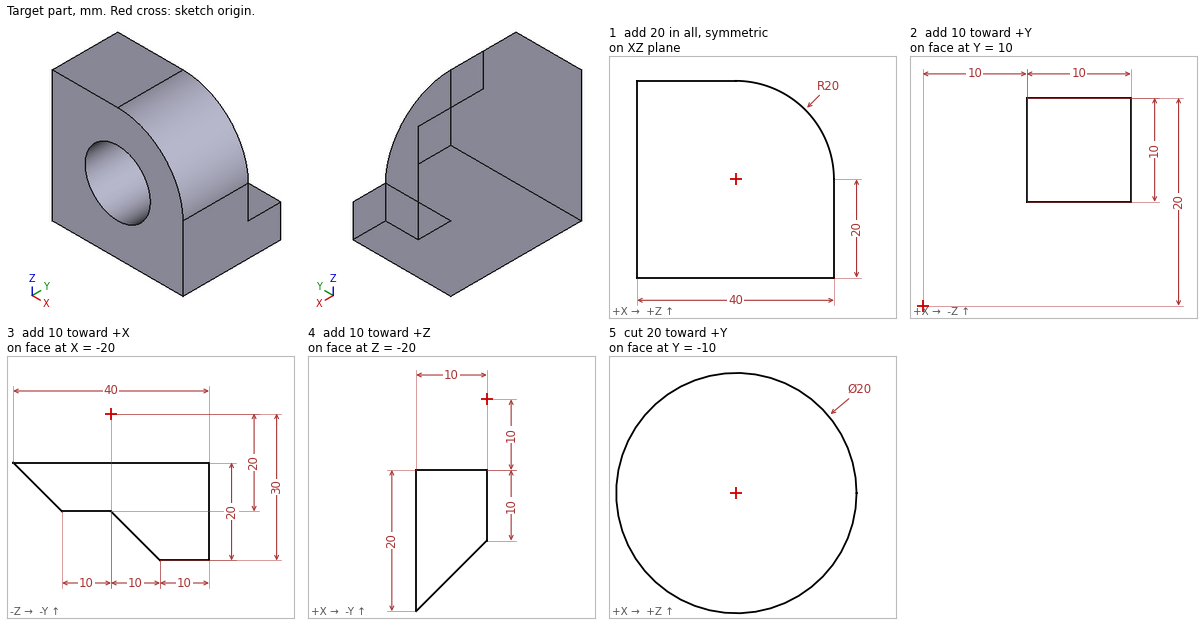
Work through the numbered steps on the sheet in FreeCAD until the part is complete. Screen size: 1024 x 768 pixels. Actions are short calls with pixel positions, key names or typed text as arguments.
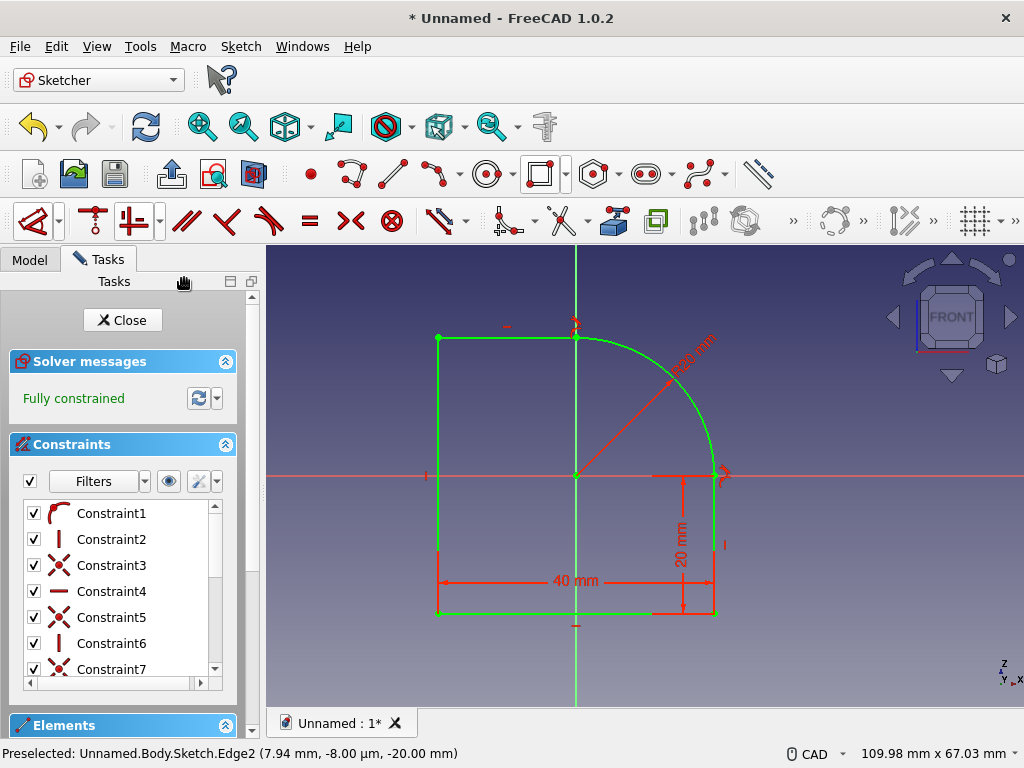
click(123, 320)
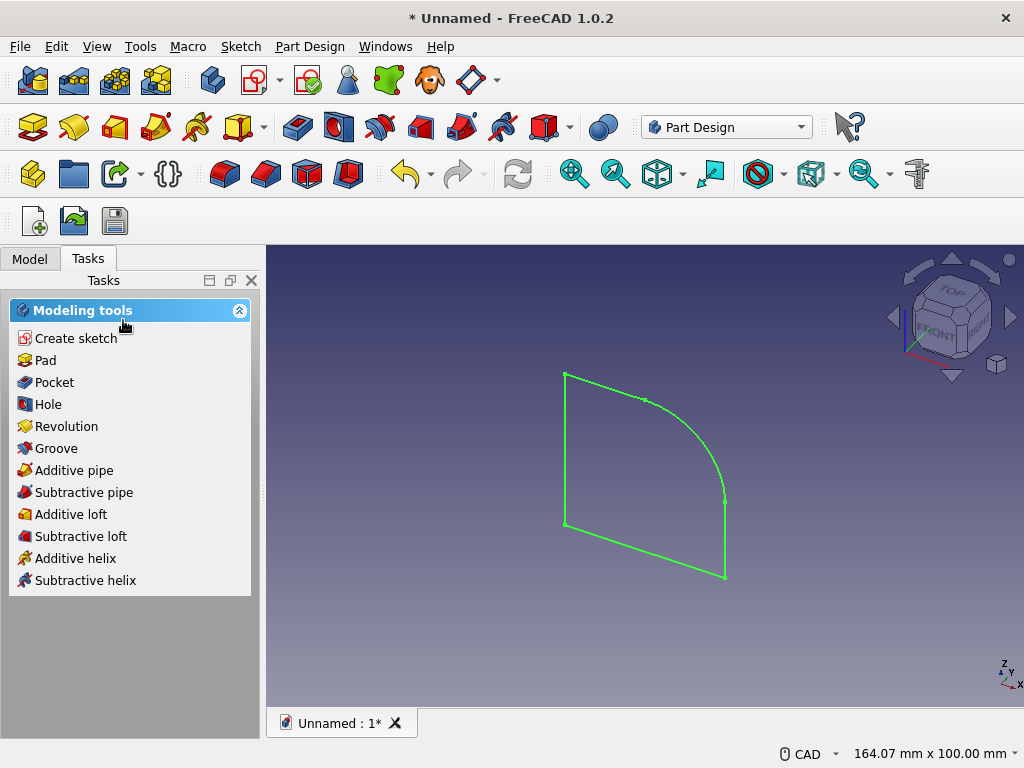
click(33, 128)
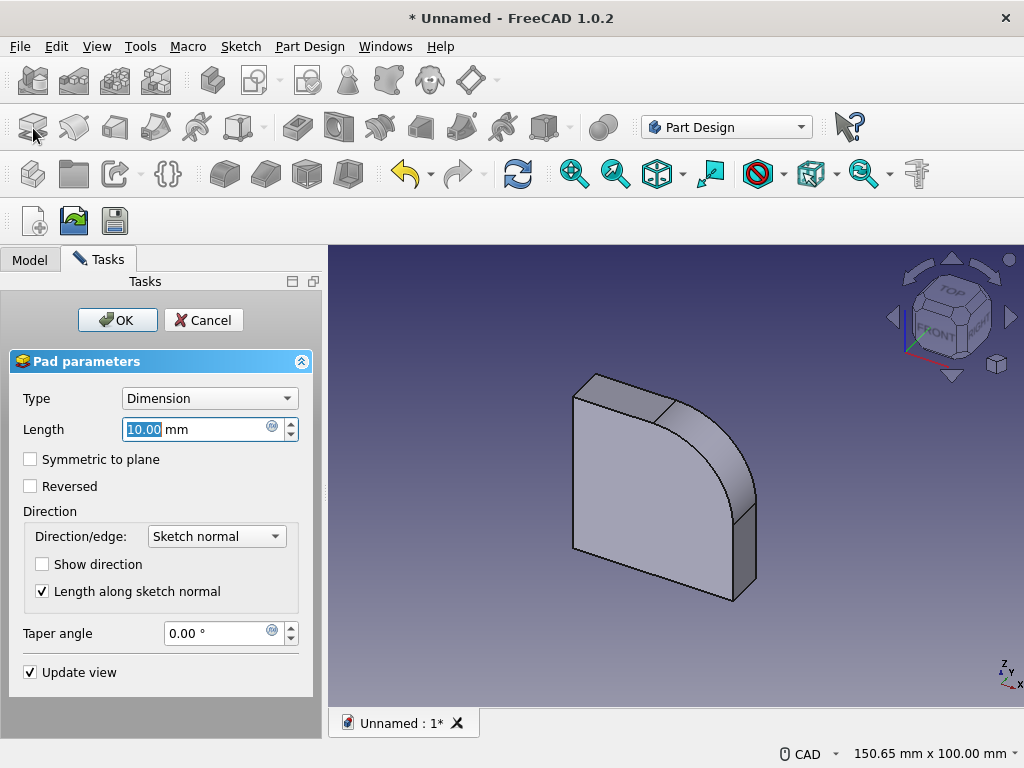
text(20)
key(Tab)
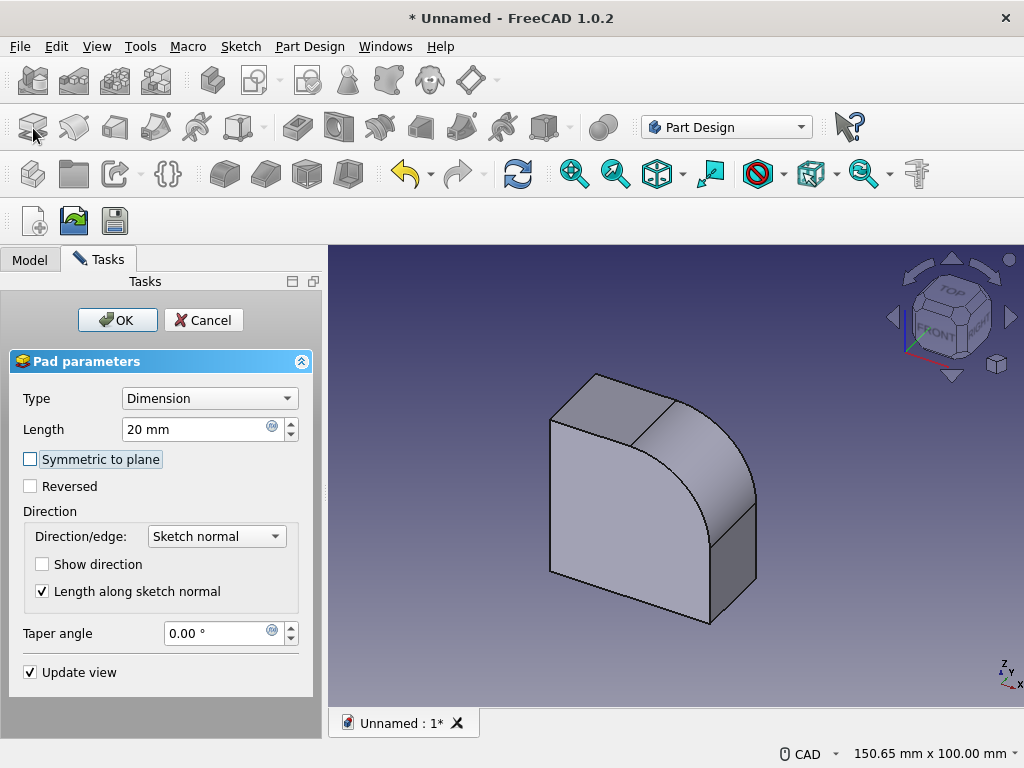
click(31, 459)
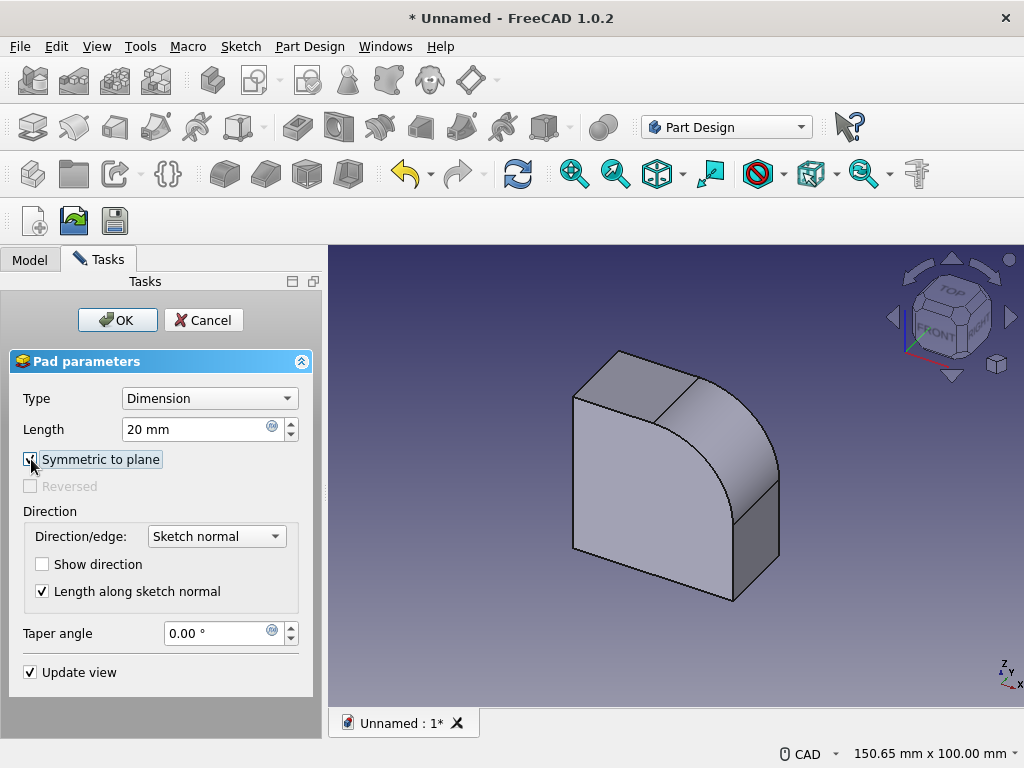
click(118, 320)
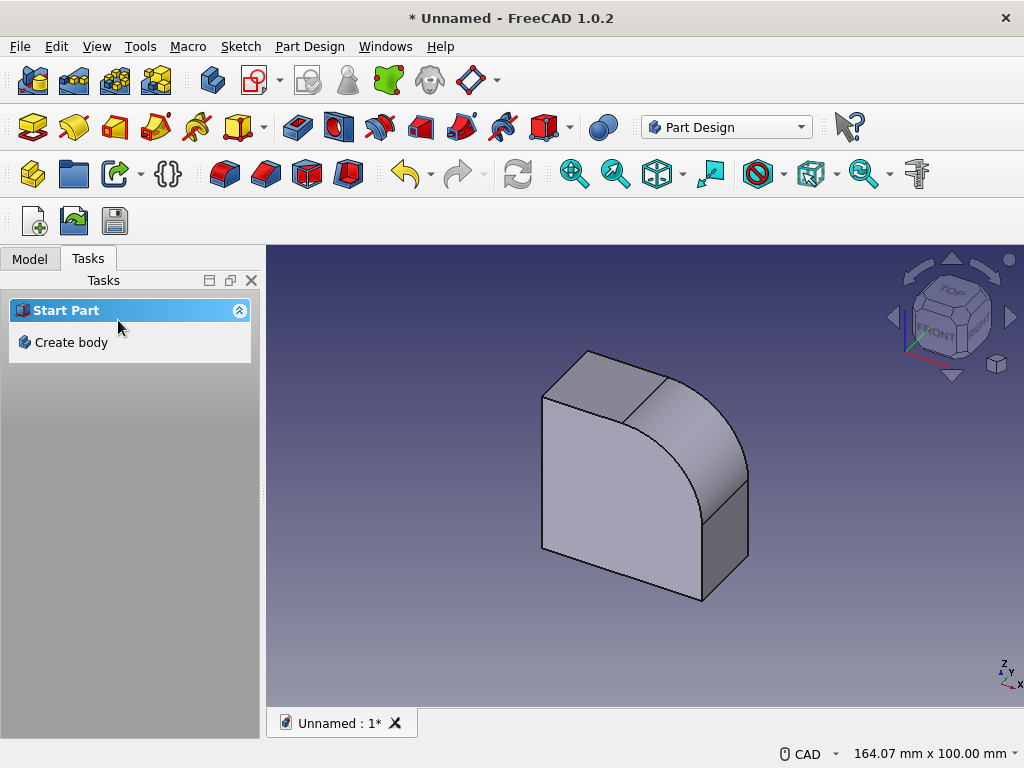
key(4)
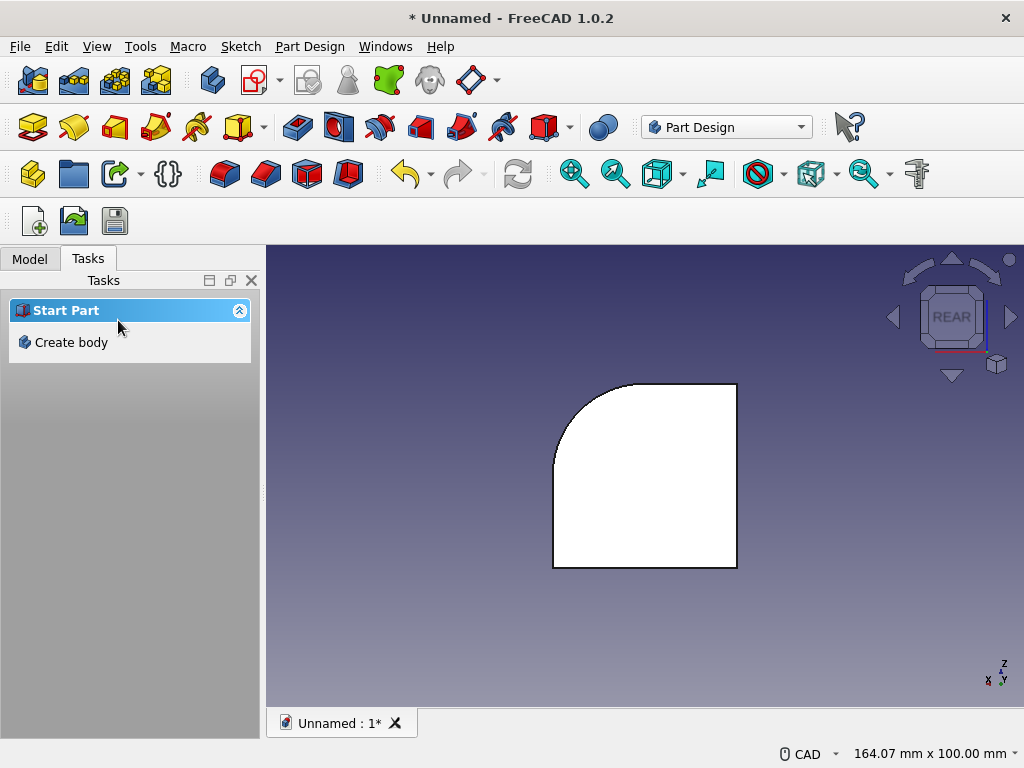
click(575, 174)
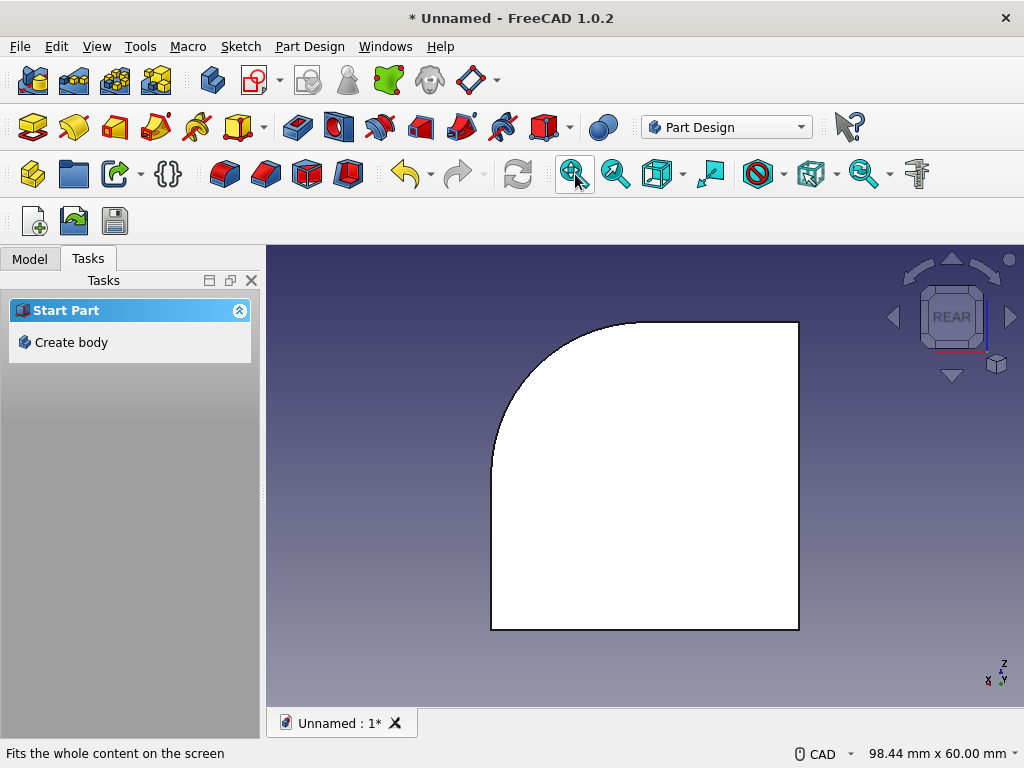
click(645, 475)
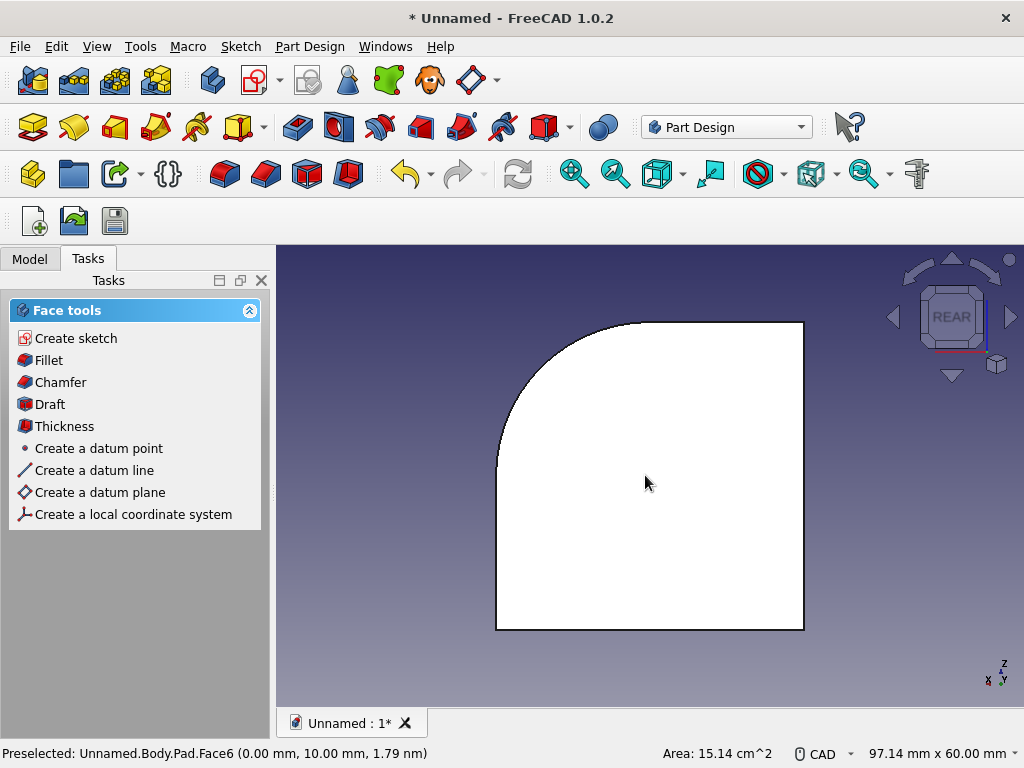
click(254, 80)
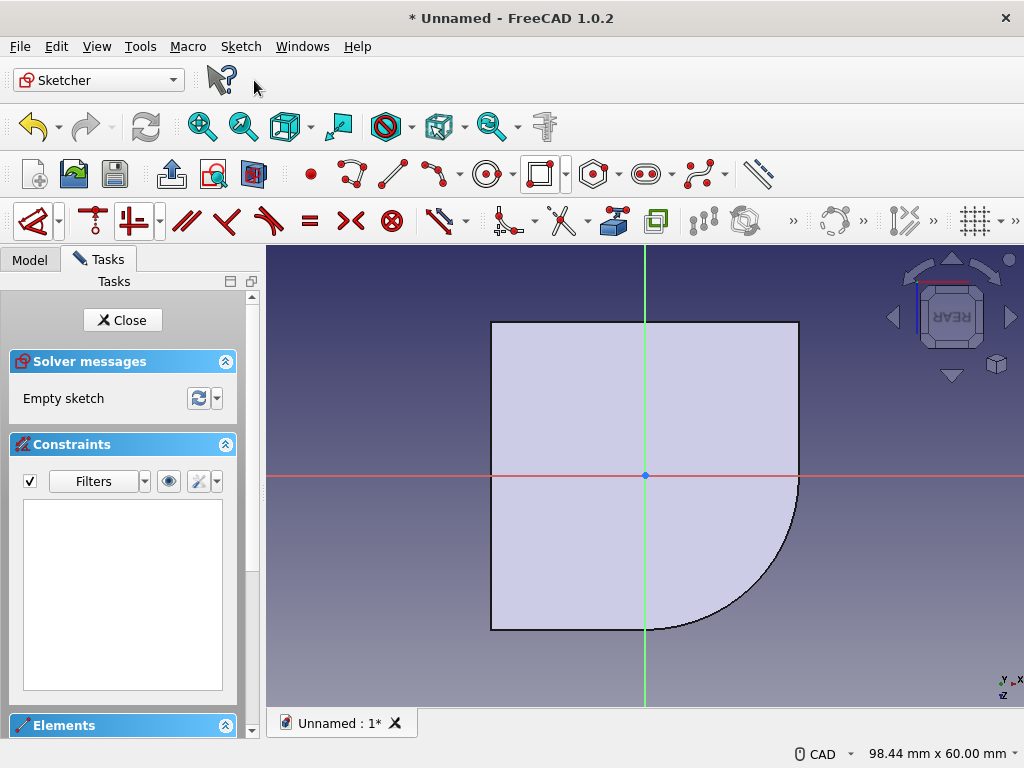
scroll(859, 305, up, 3)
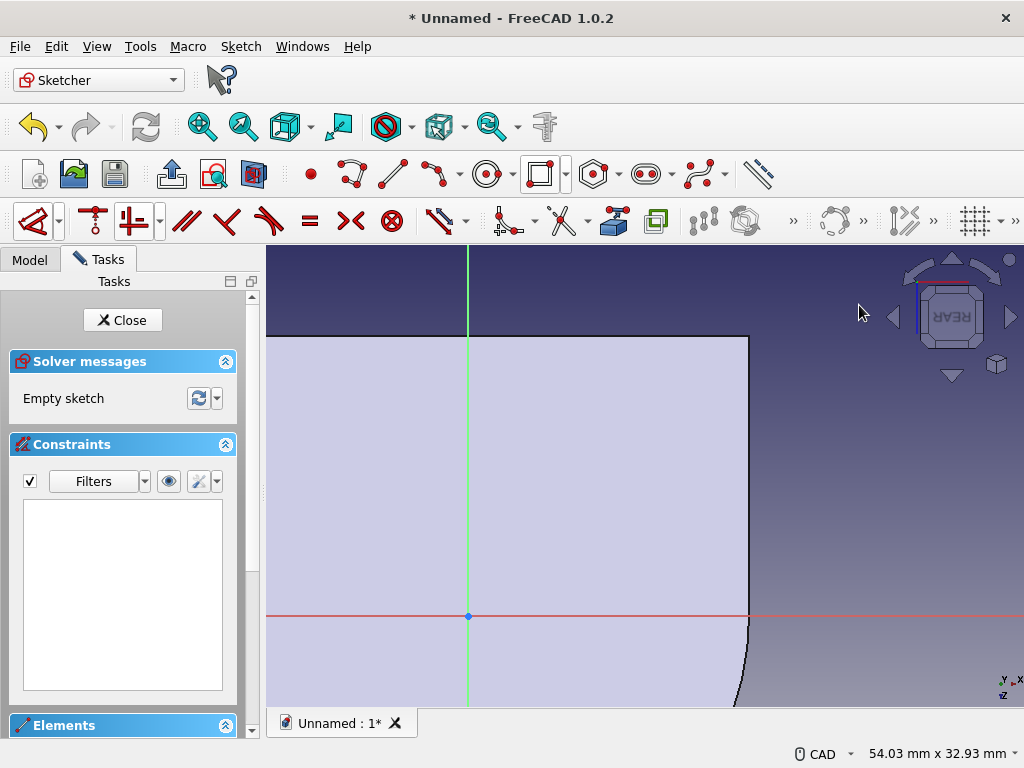
click(540, 174)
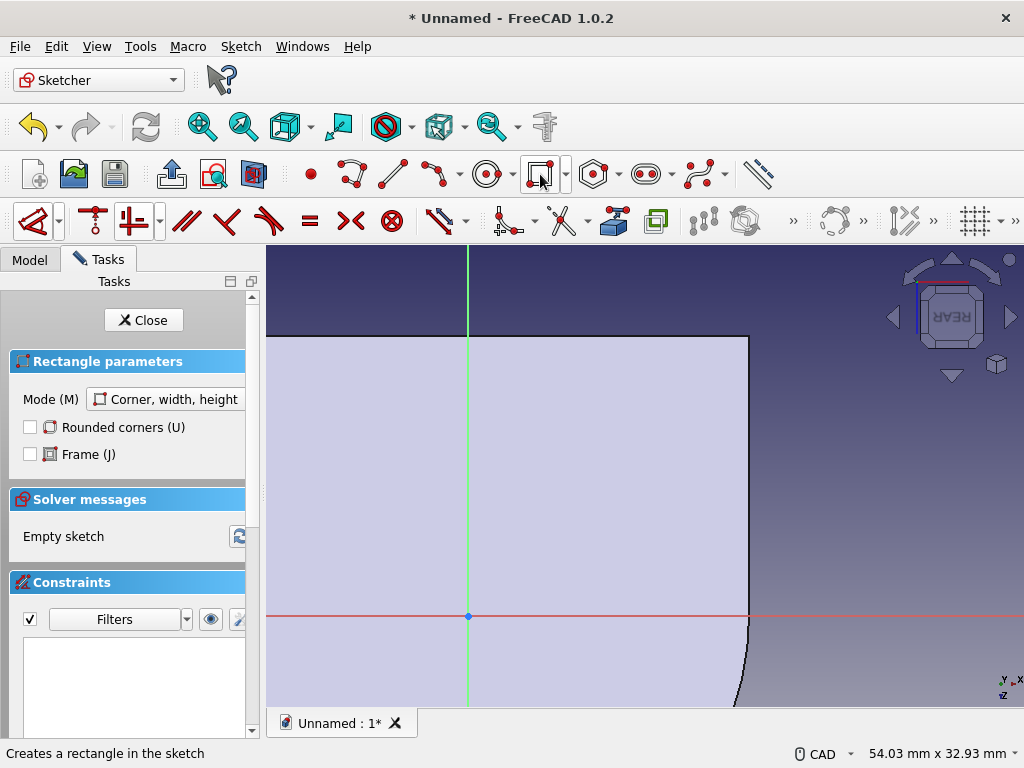
click(609, 336)
click(749, 476)
key(Escape)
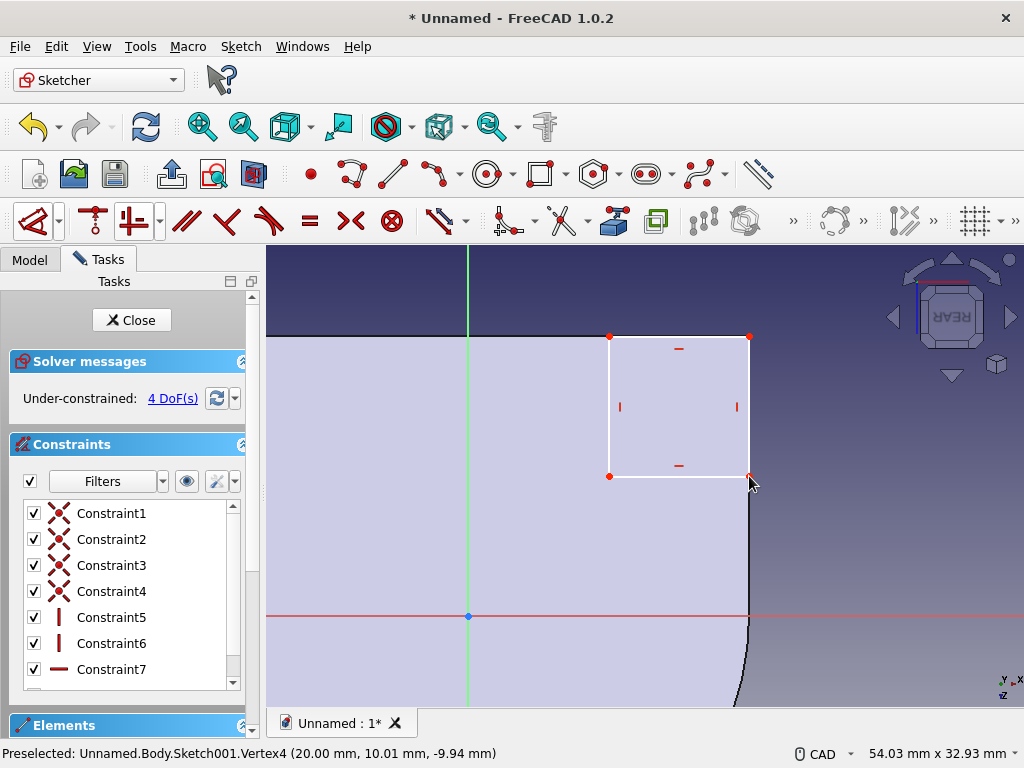
click(609, 379)